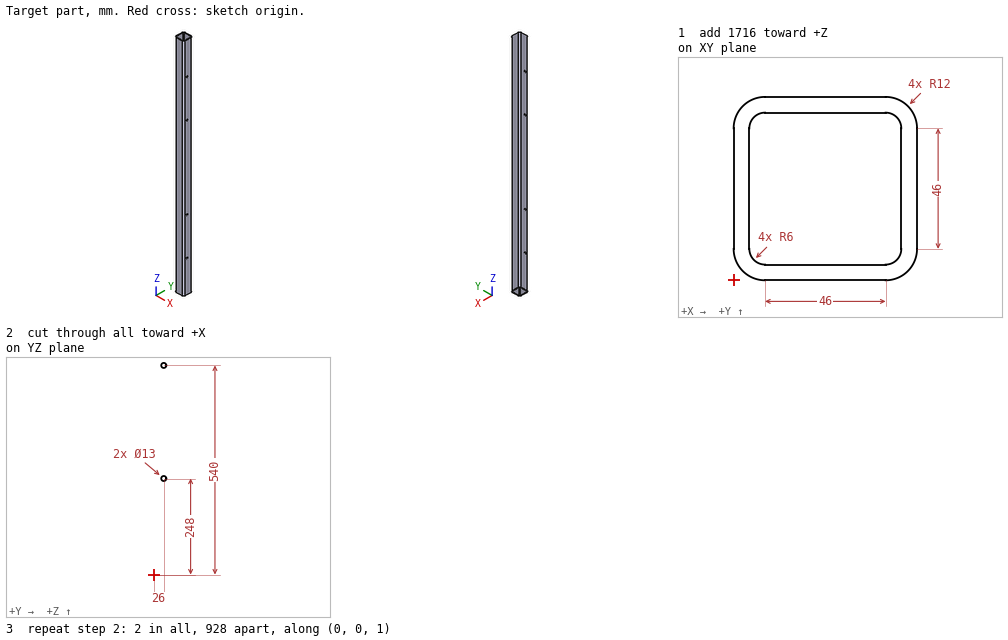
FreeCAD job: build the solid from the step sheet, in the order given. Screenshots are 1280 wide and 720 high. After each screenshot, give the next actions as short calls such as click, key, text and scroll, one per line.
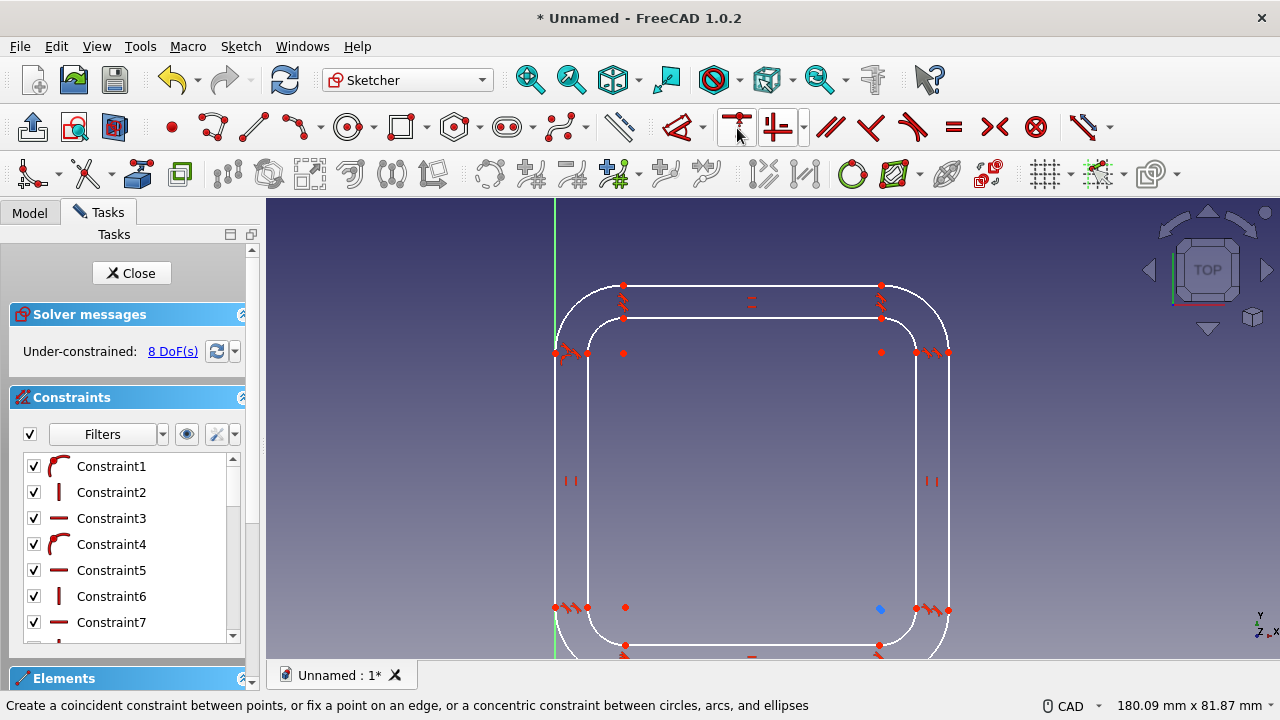
scroll(607, 322, down, 2)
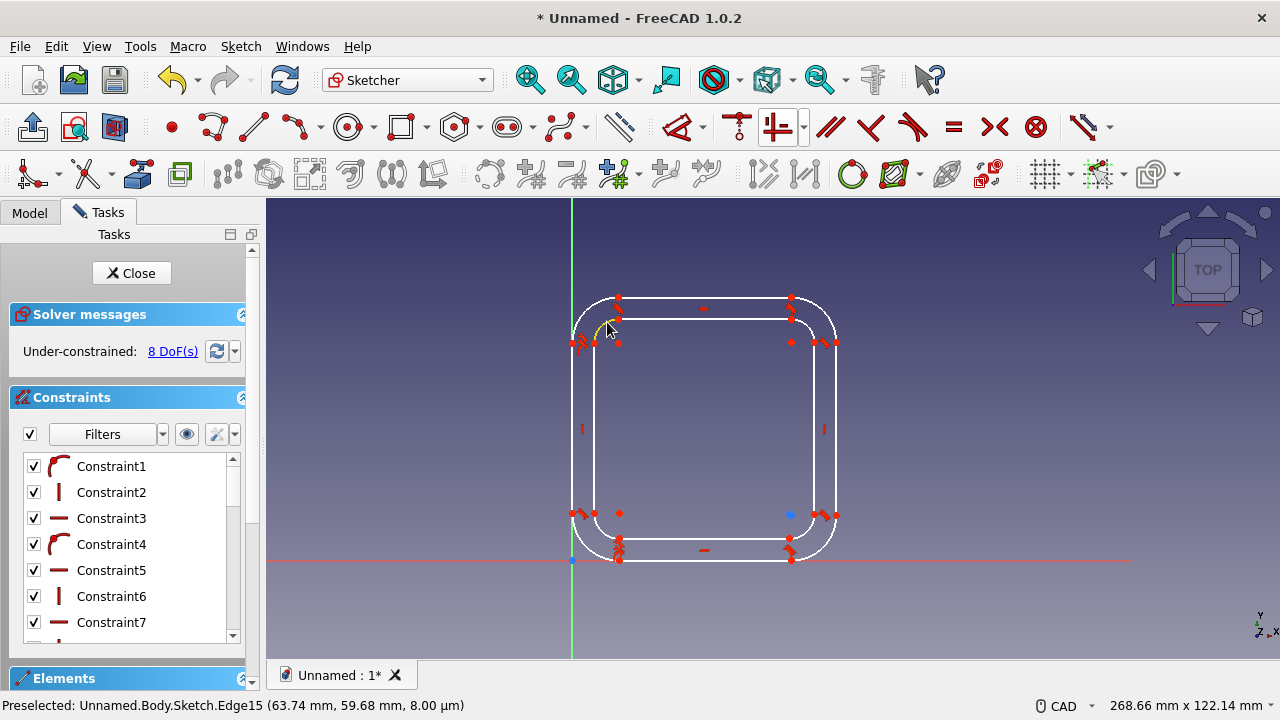
click(831, 536)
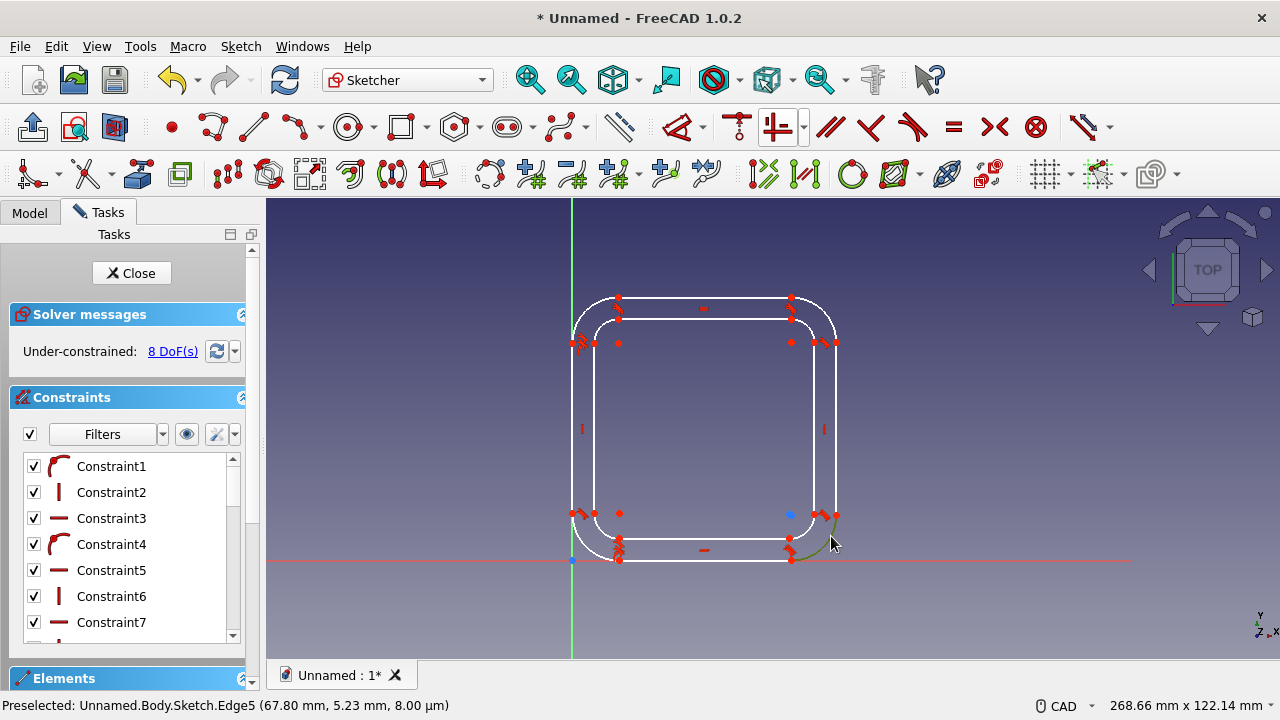
click(831, 322)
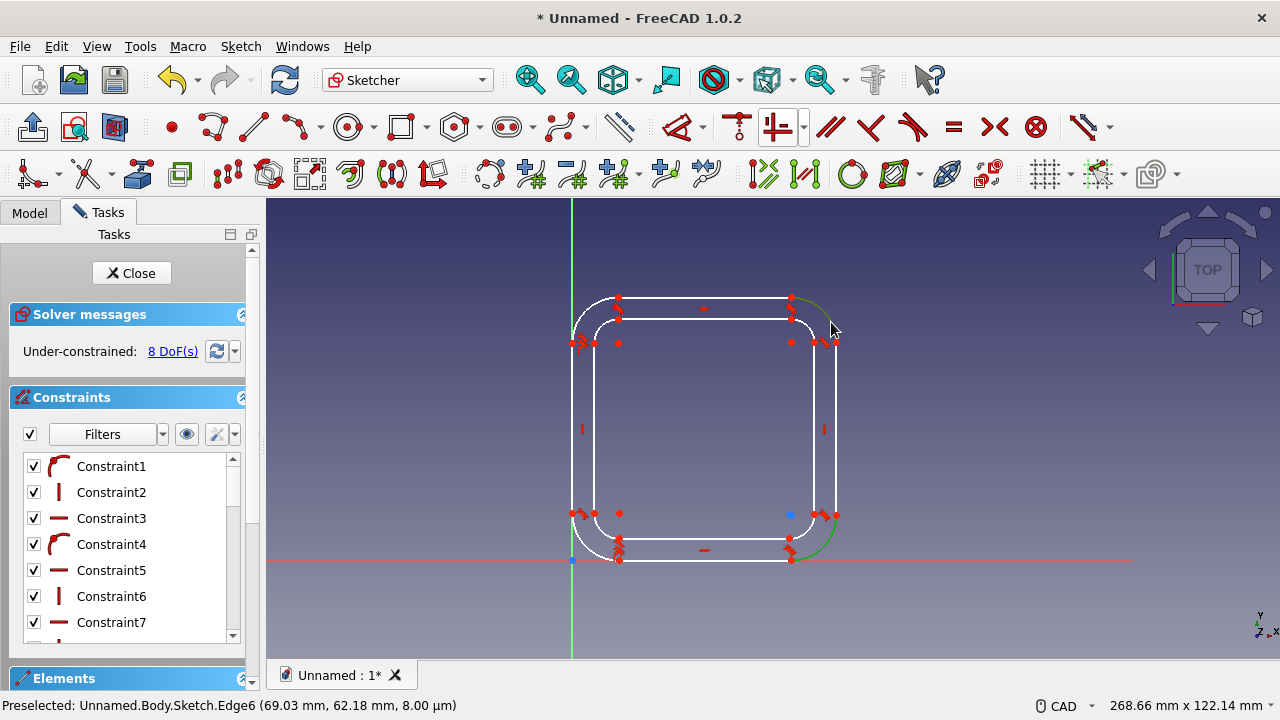
click(597, 303)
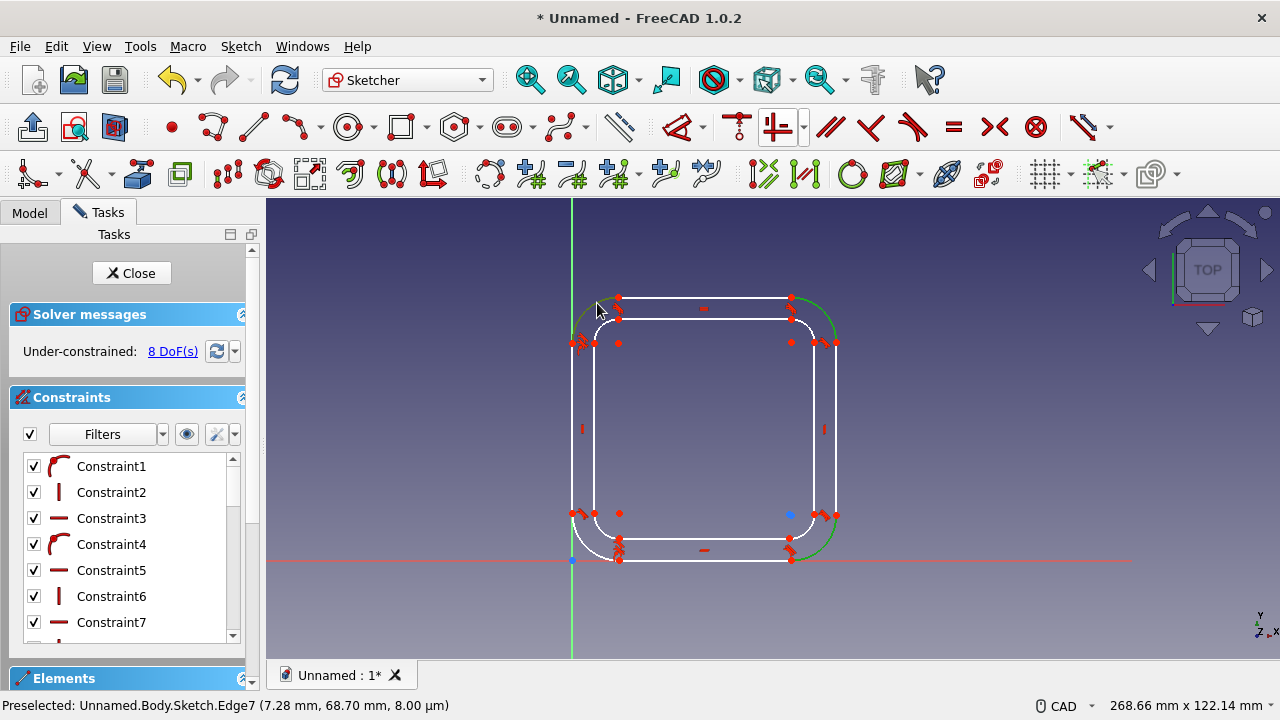
click(586, 547)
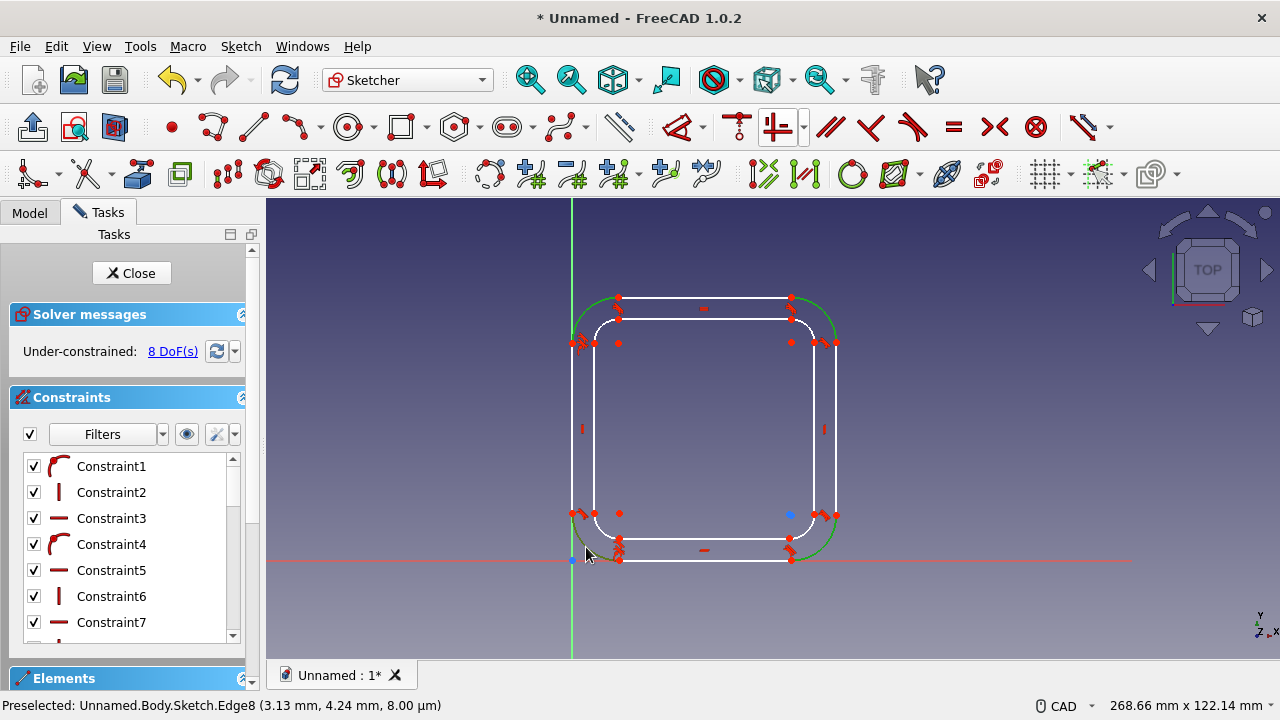
click(954, 128)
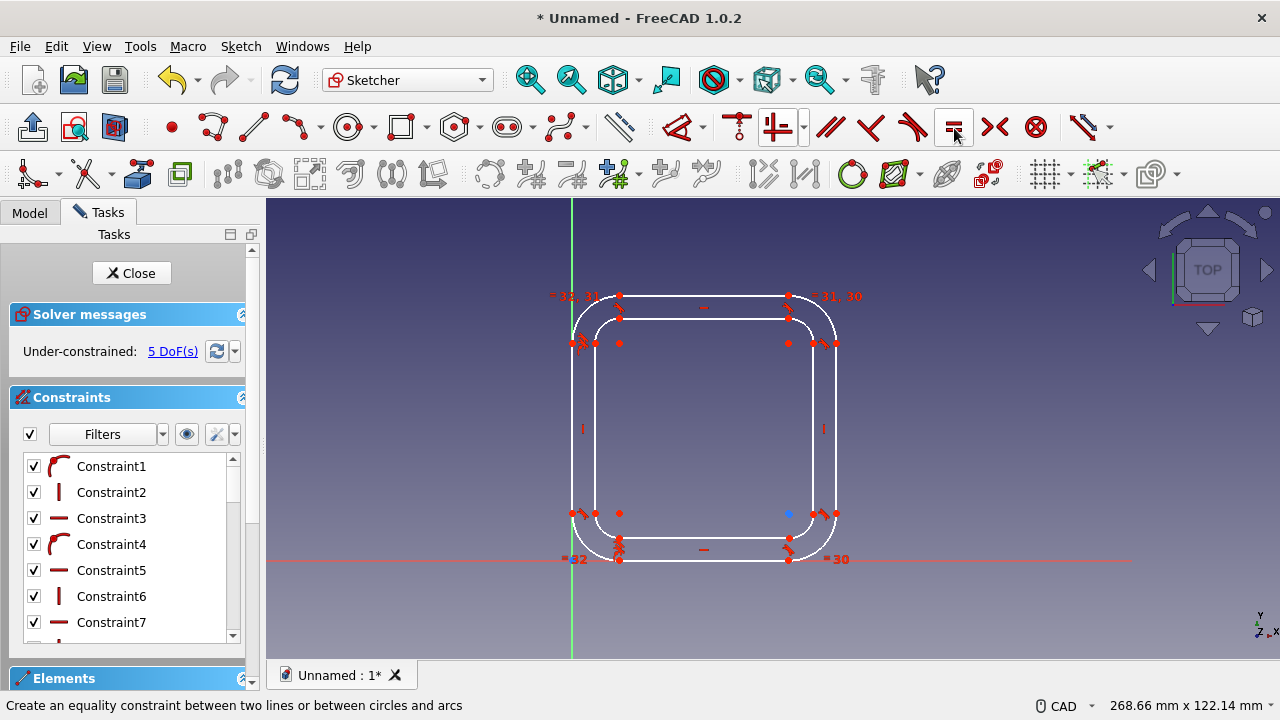
click(598, 525)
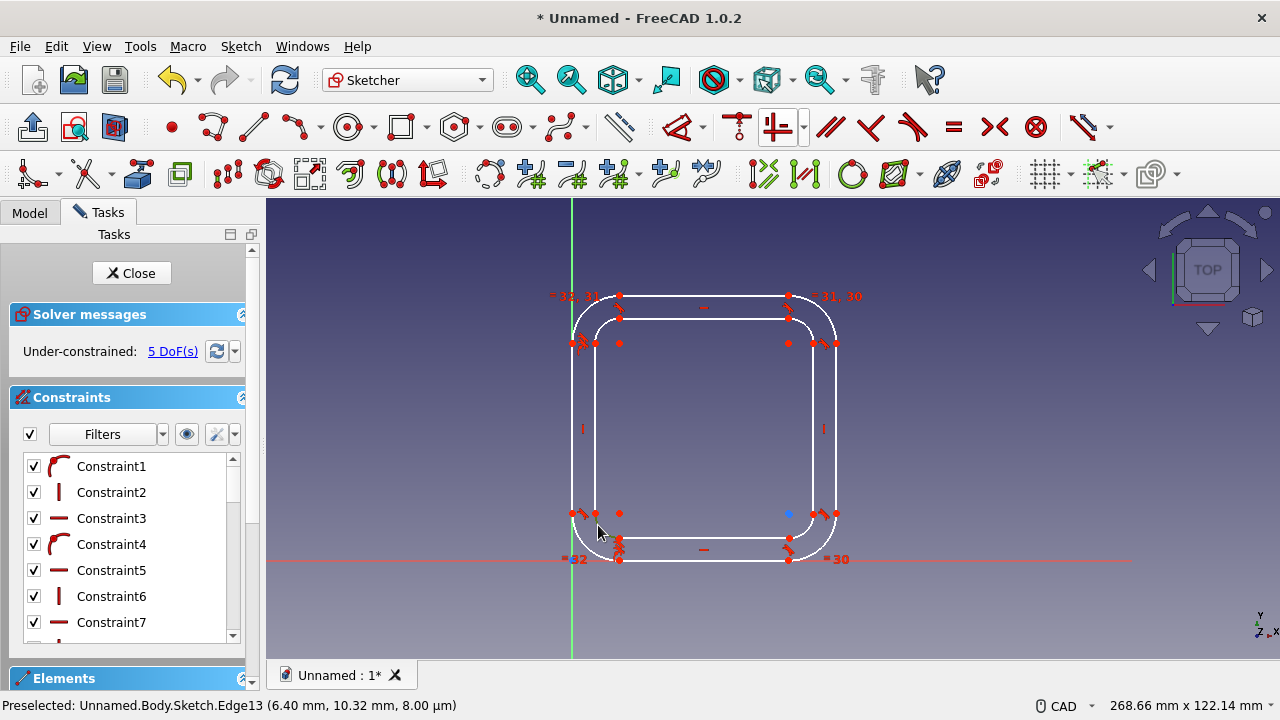
scroll(800, 535, up, 2)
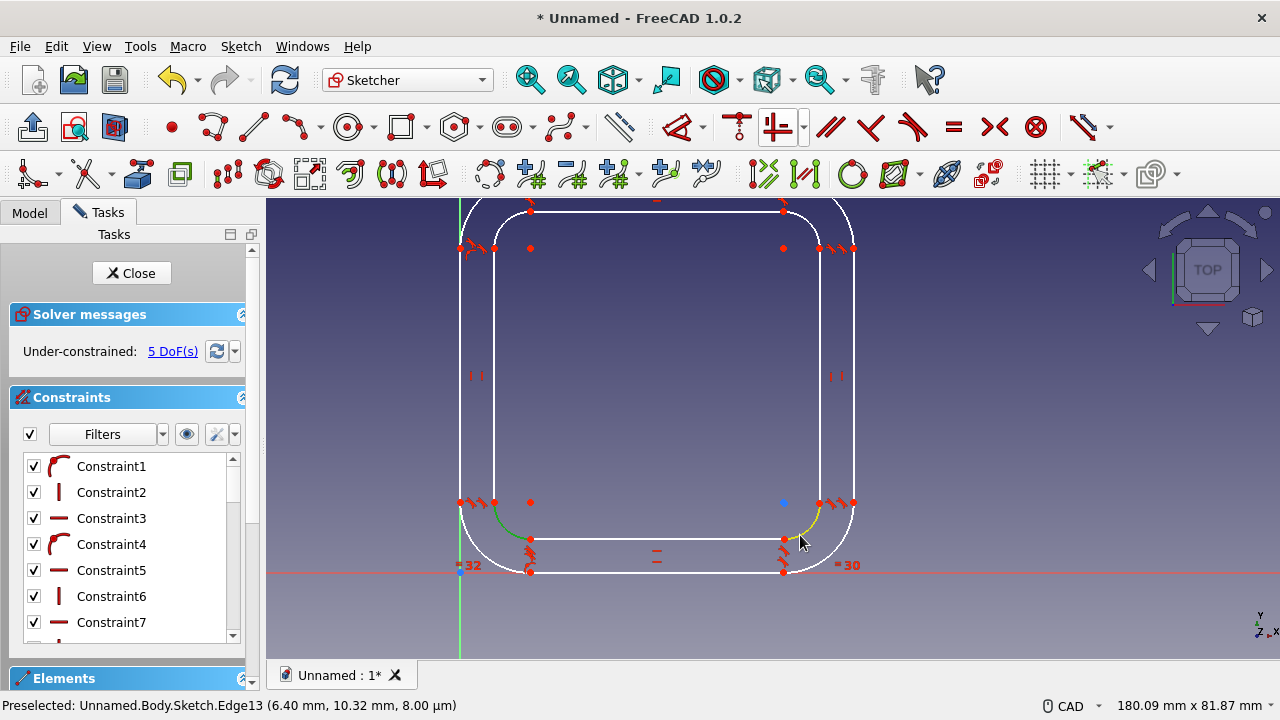
click(800, 535)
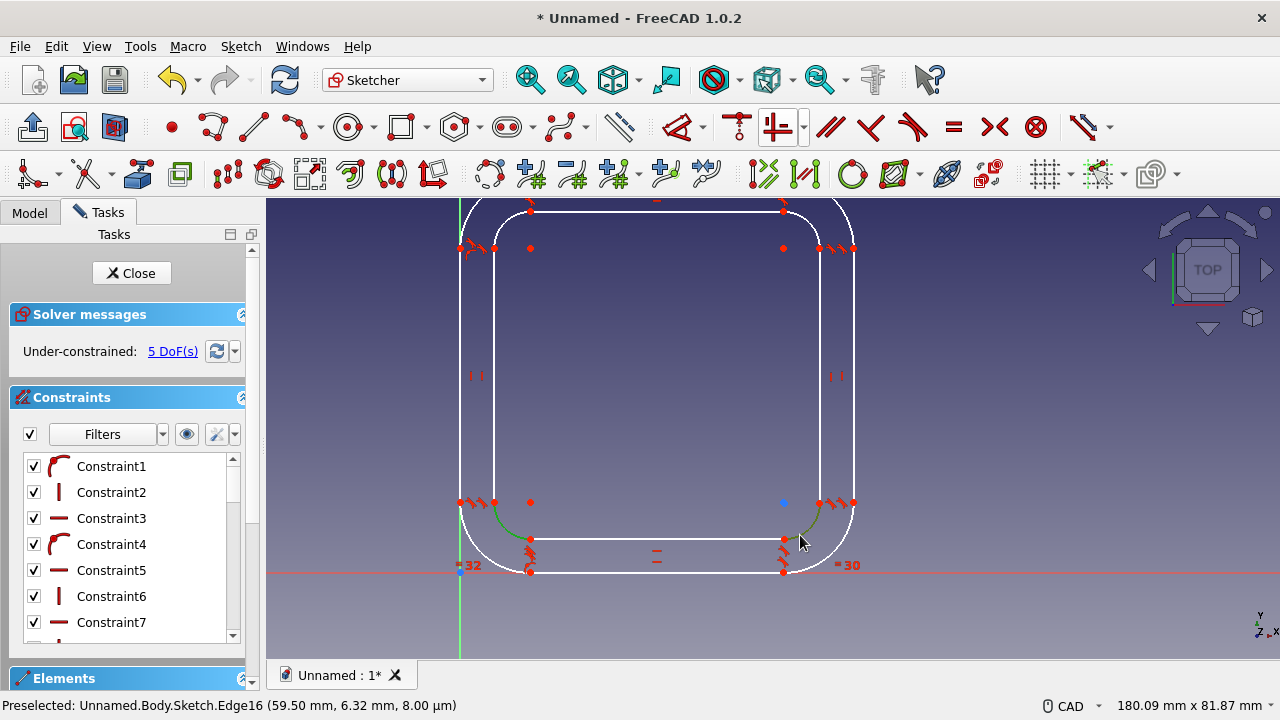
click(954, 128)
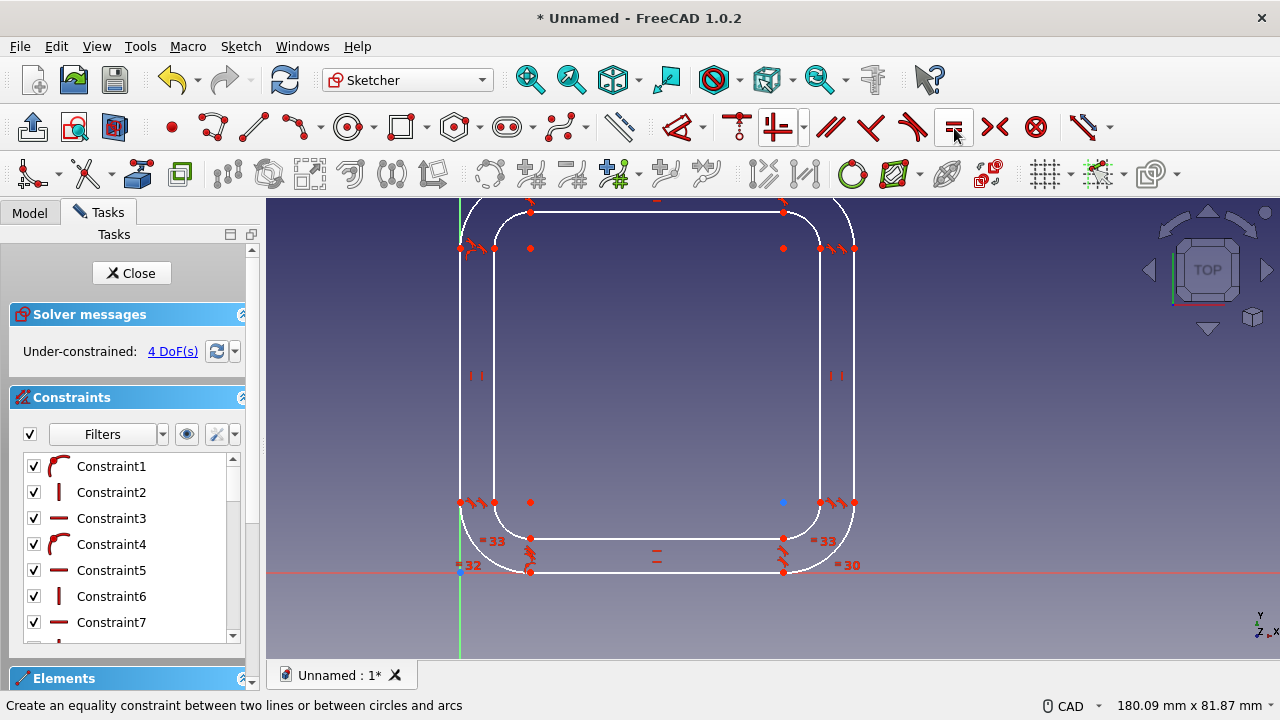
click(847, 534)